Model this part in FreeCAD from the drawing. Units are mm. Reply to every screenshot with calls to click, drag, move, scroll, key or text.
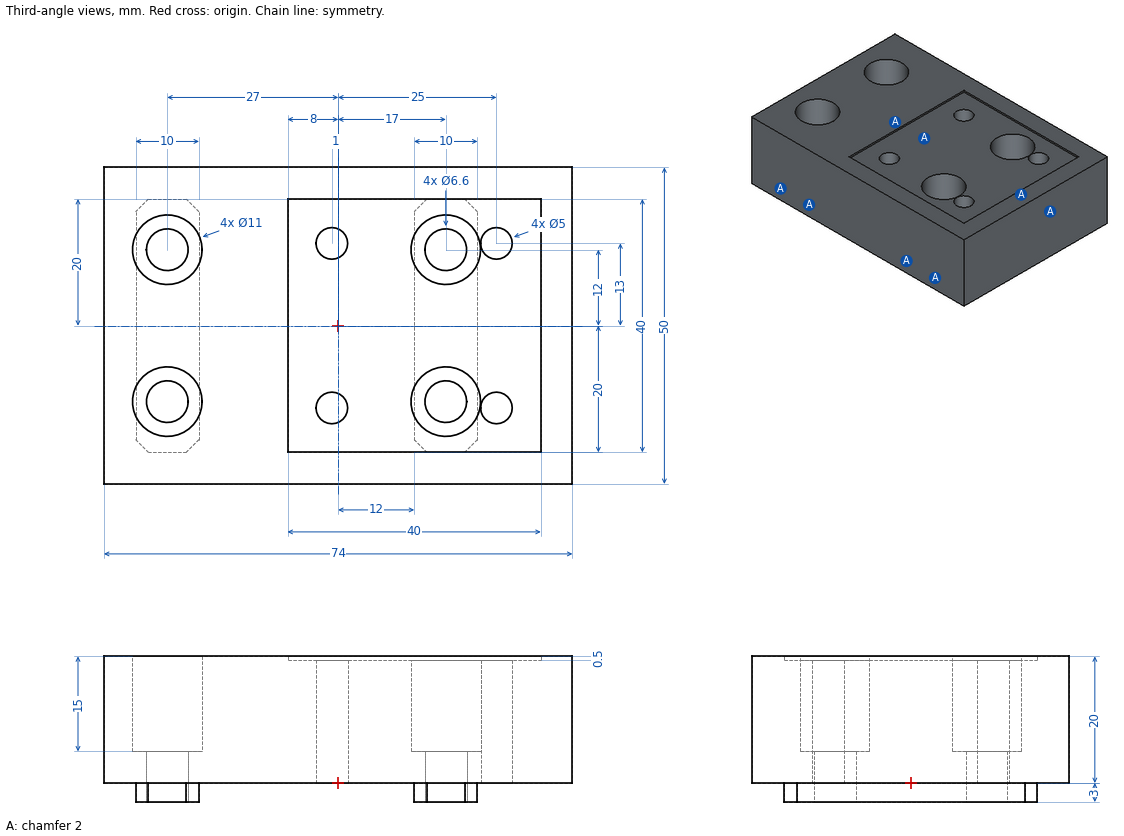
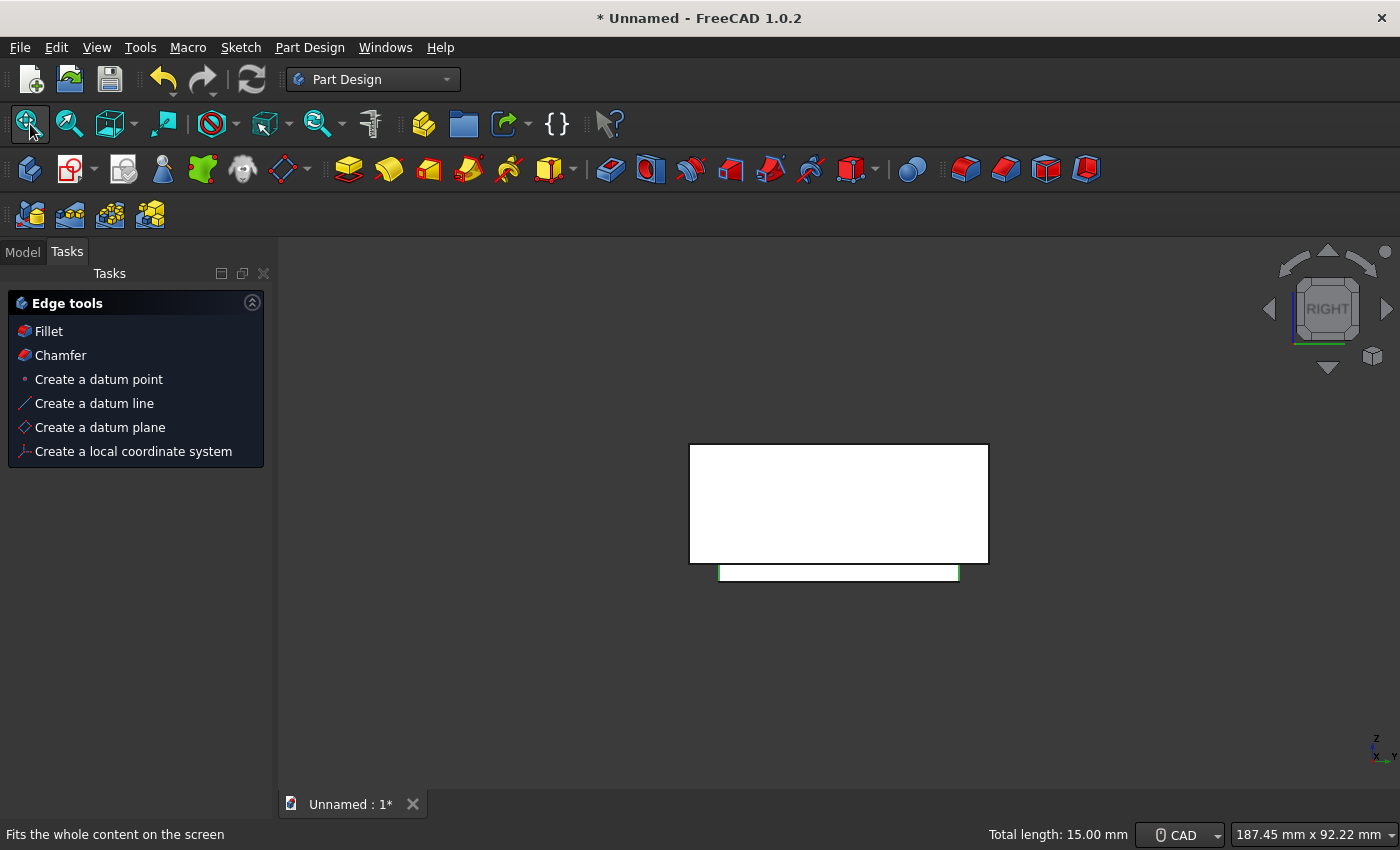
scroll(911, 632, up, 5)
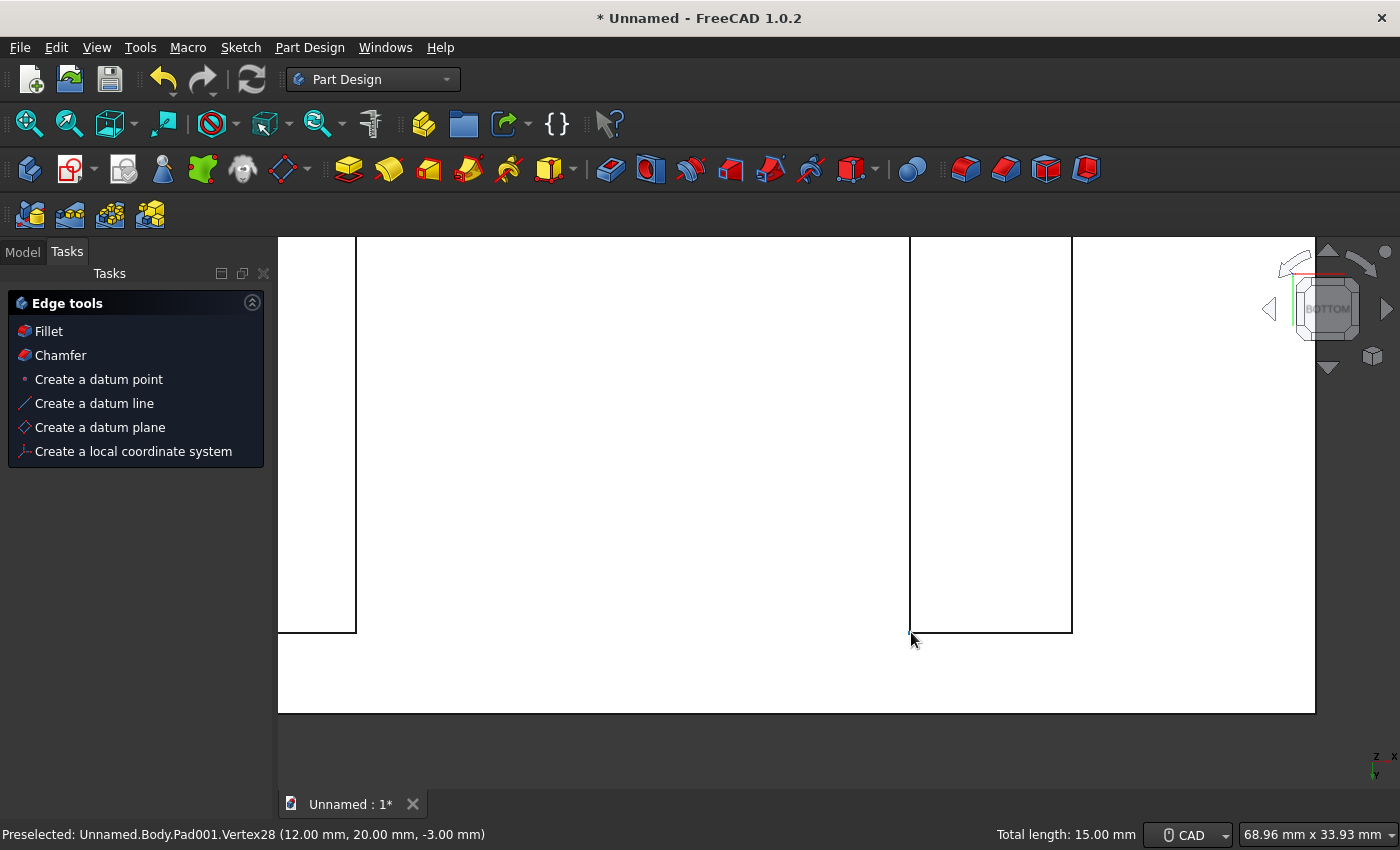
click(30, 124)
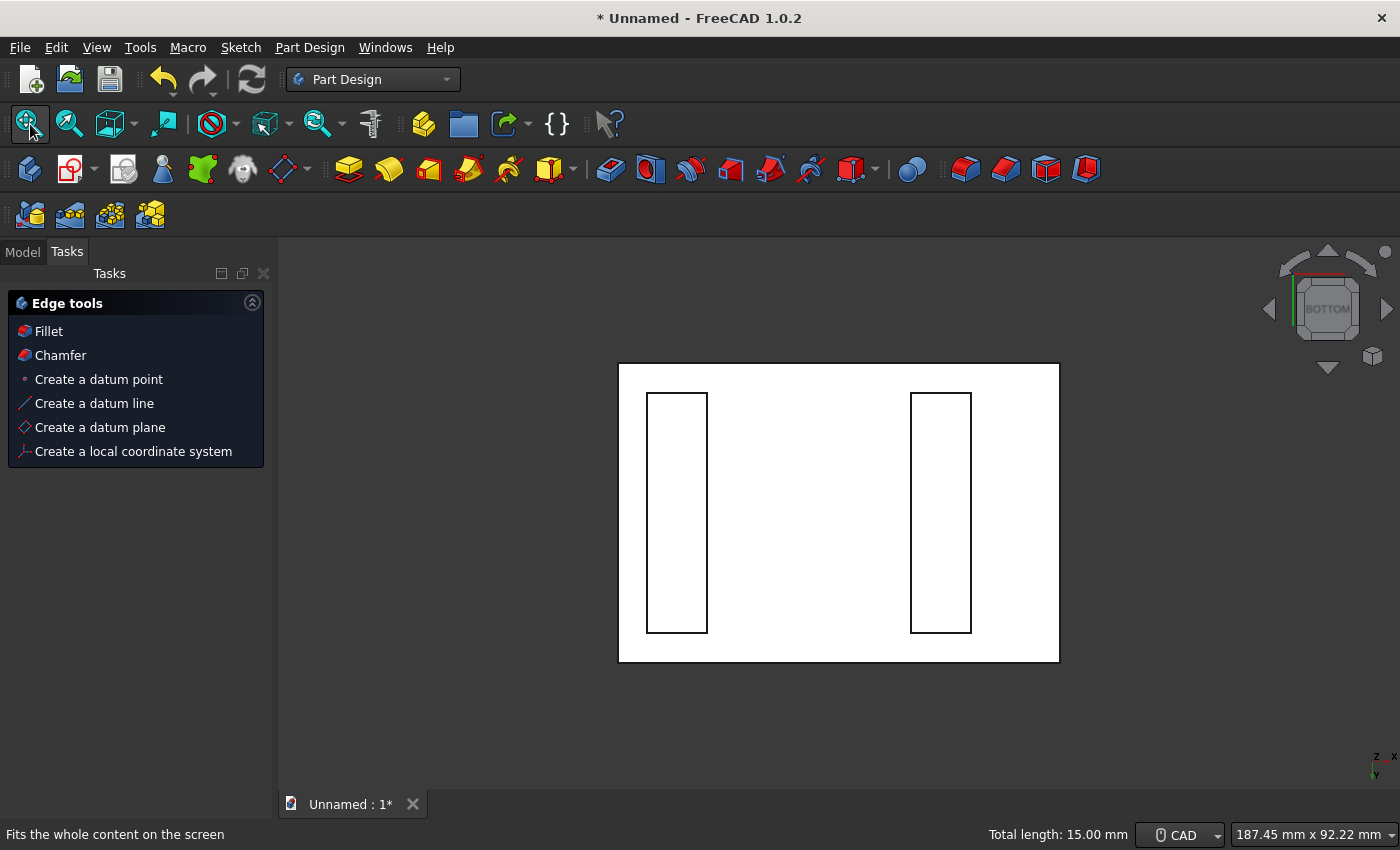
key(4)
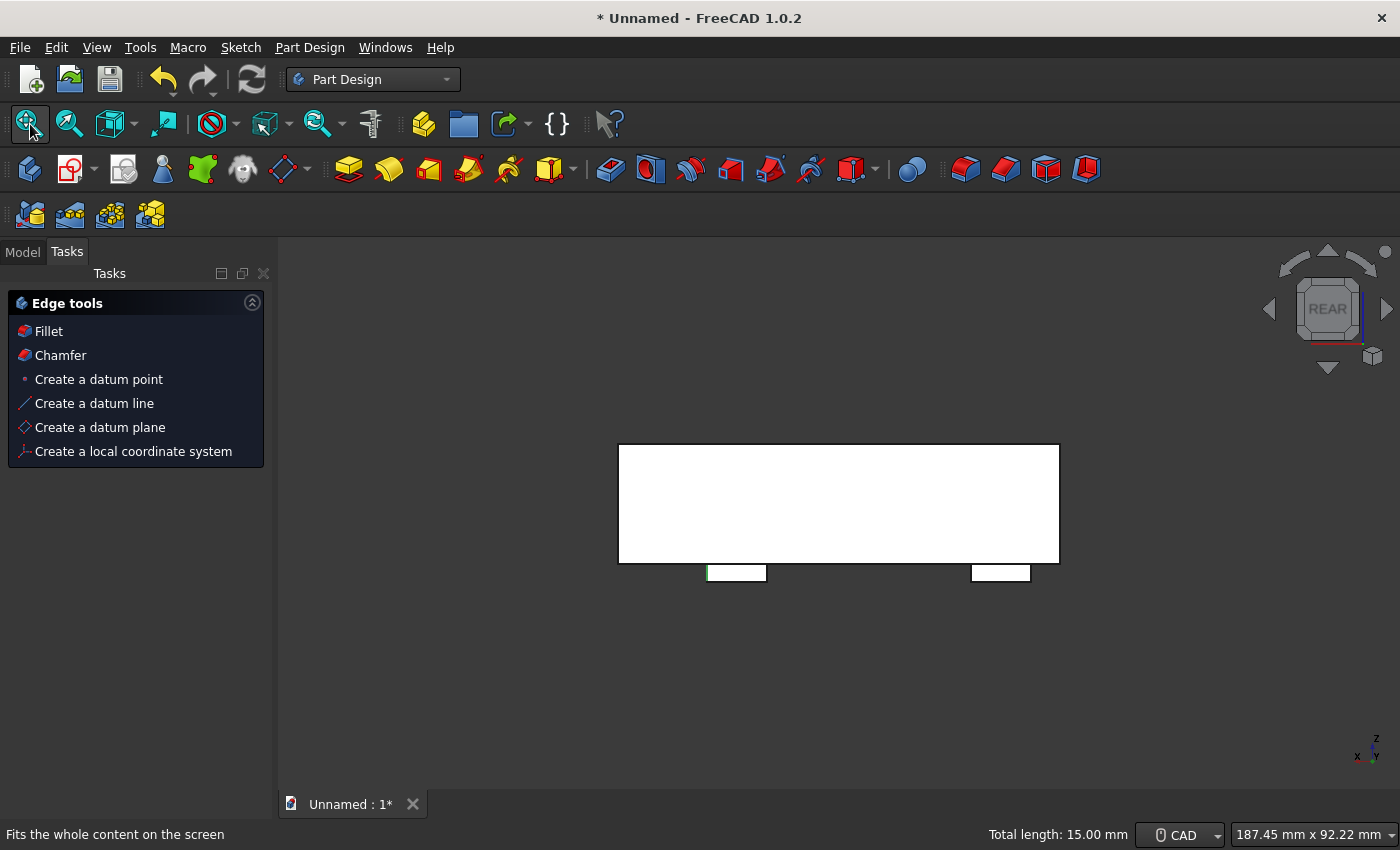
click(30, 124)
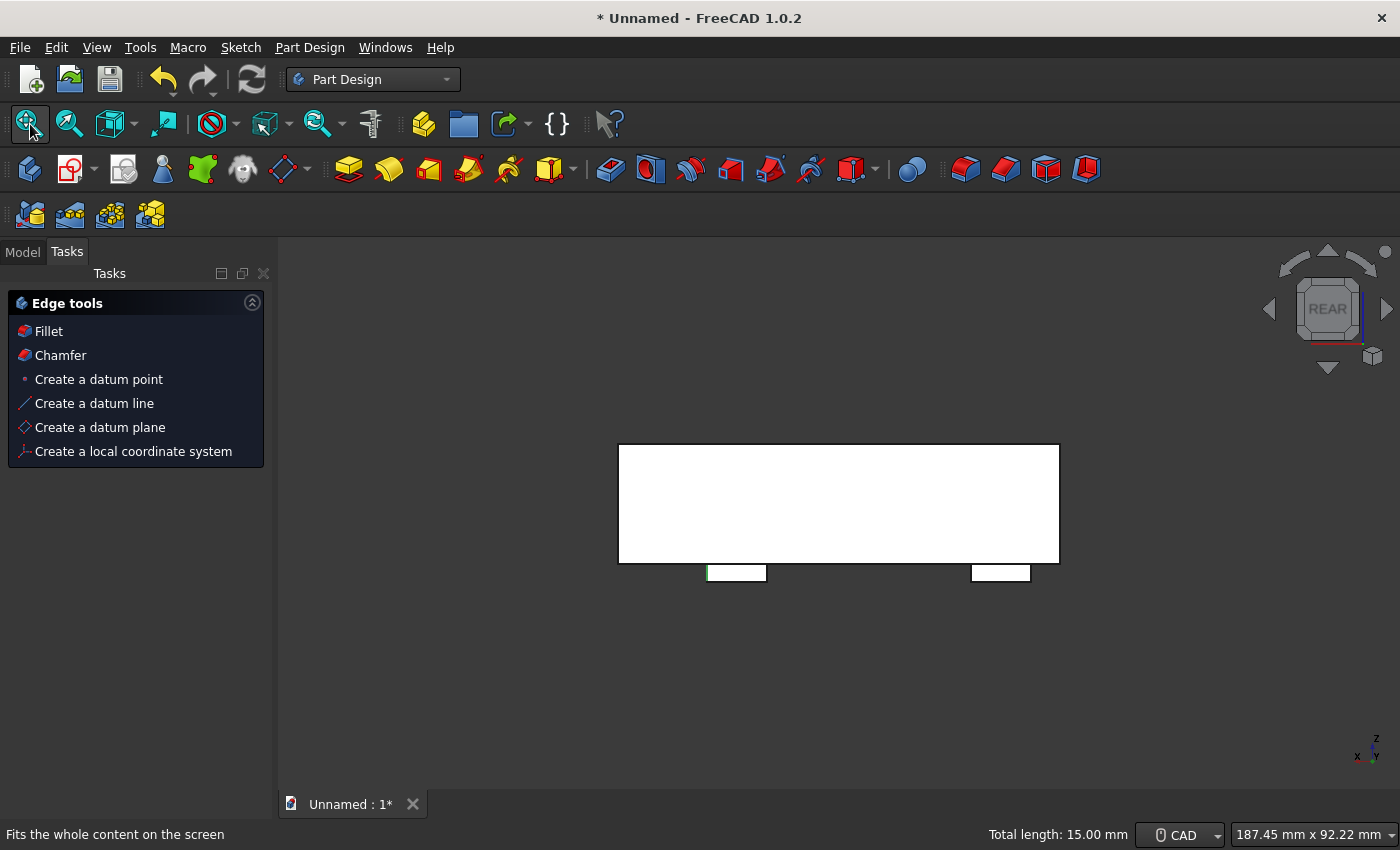
click(767, 572, ctrl)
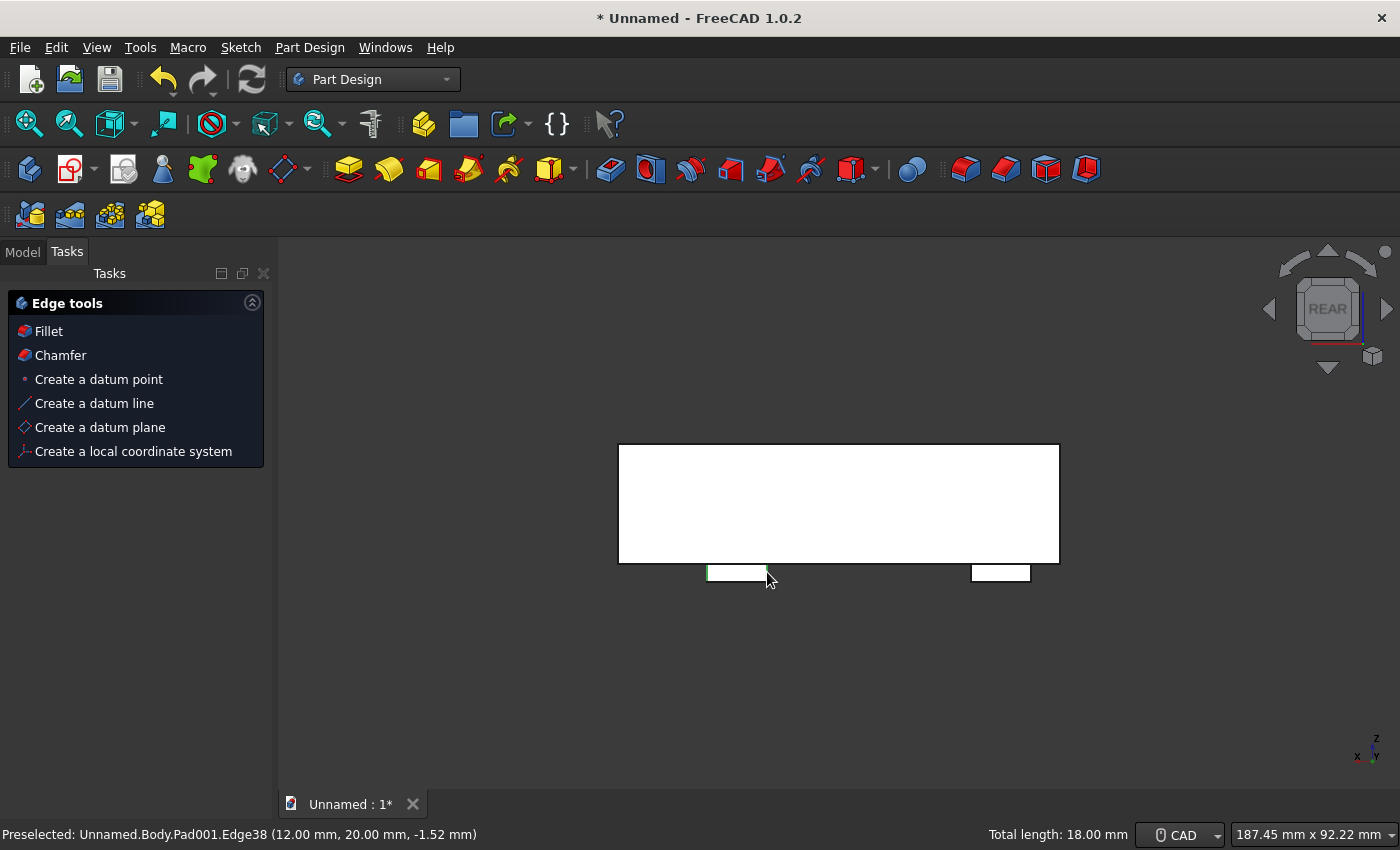
click(971, 572, ctrl)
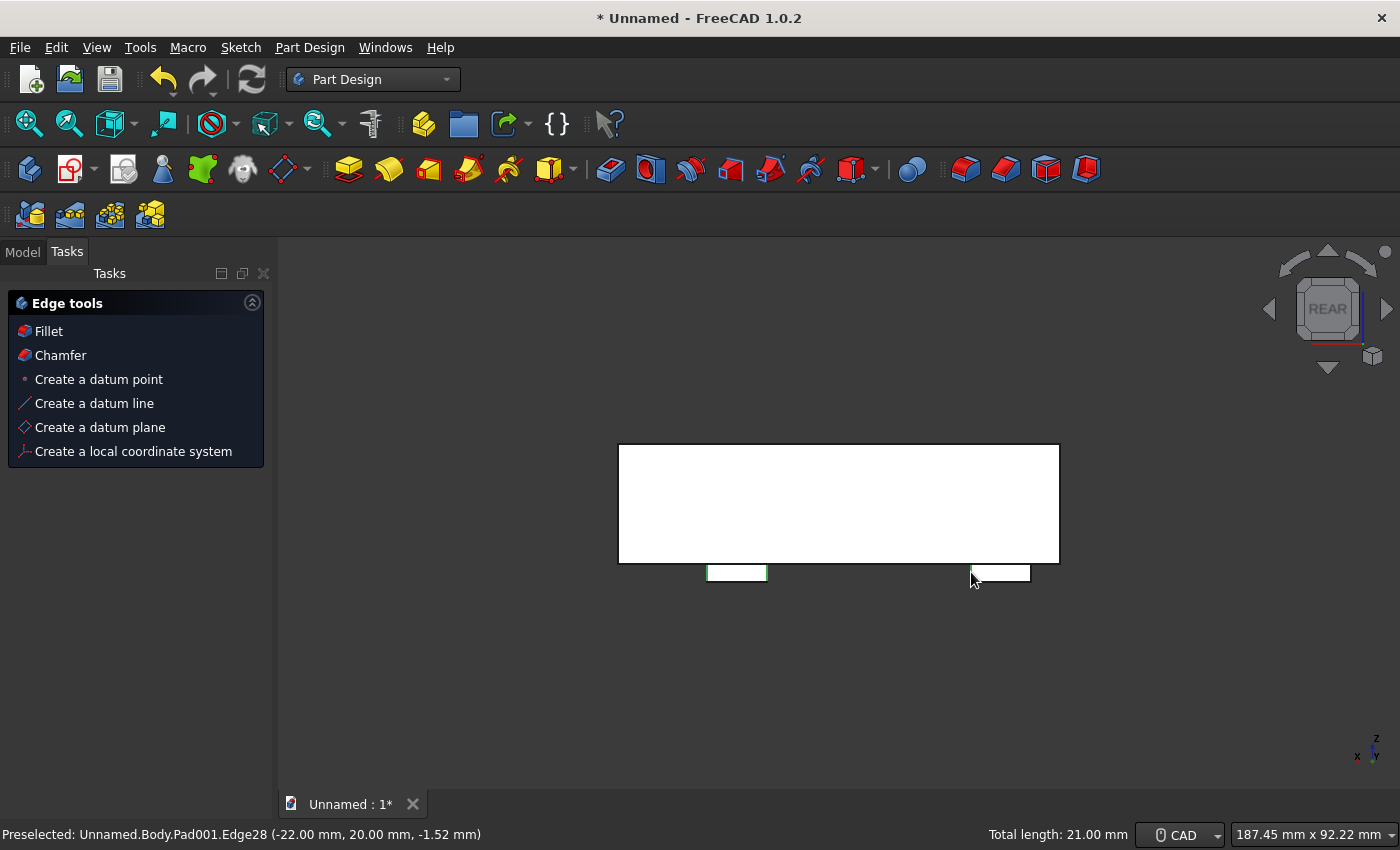
click(1031, 572, ctrl)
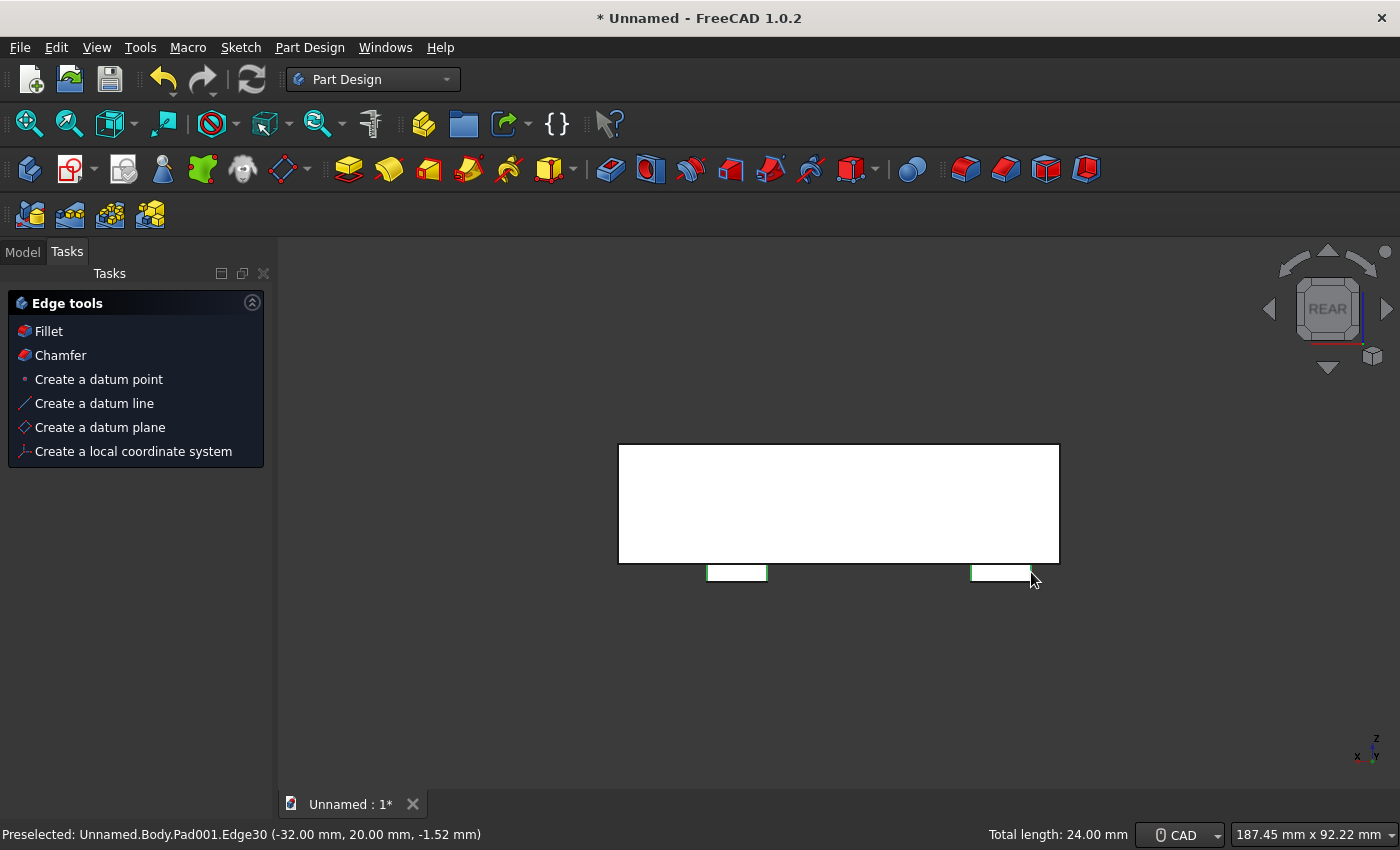
click(1006, 170)